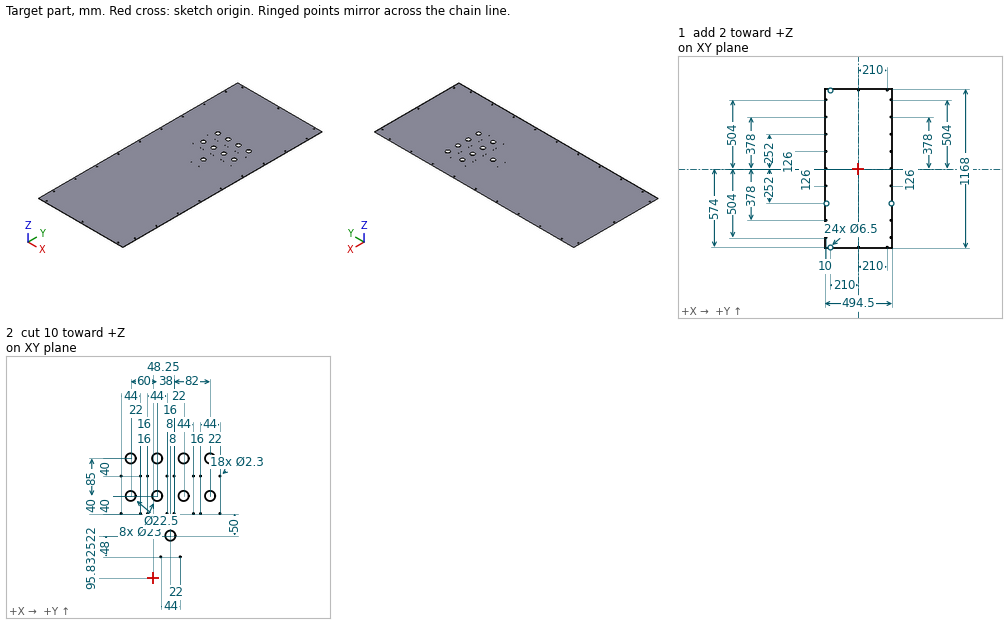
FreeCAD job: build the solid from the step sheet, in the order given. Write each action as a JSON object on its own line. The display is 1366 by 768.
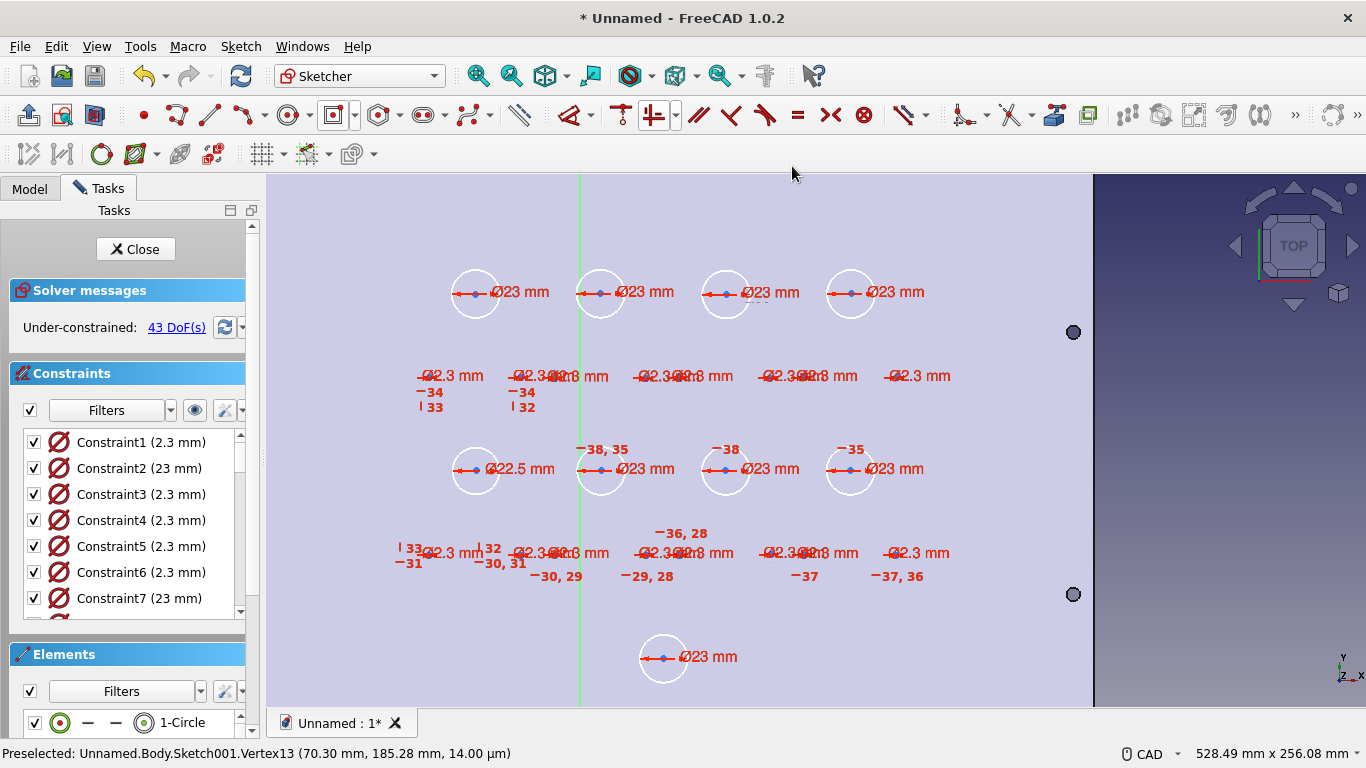
{"action": "left_click", "coordinate": [805, 555]}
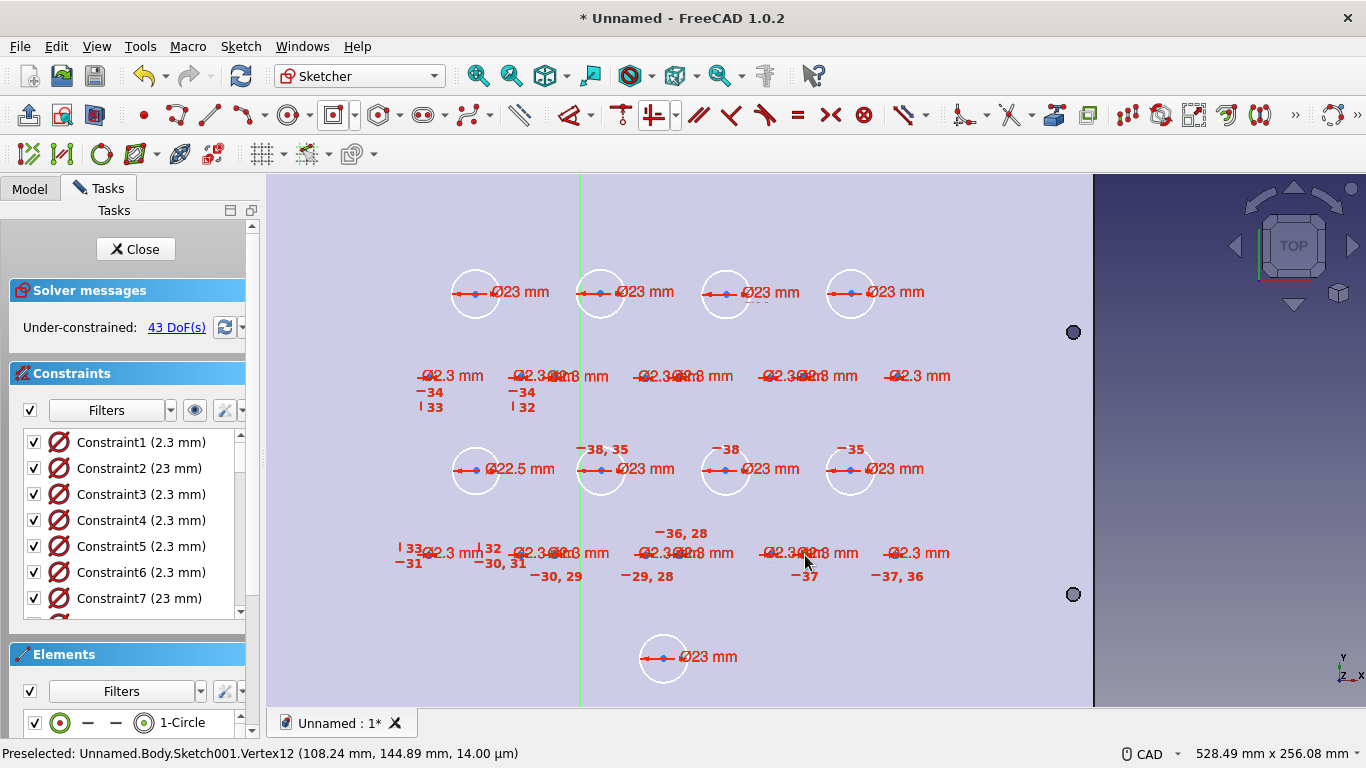
{"action": "left_click", "coordinate": [771, 555]}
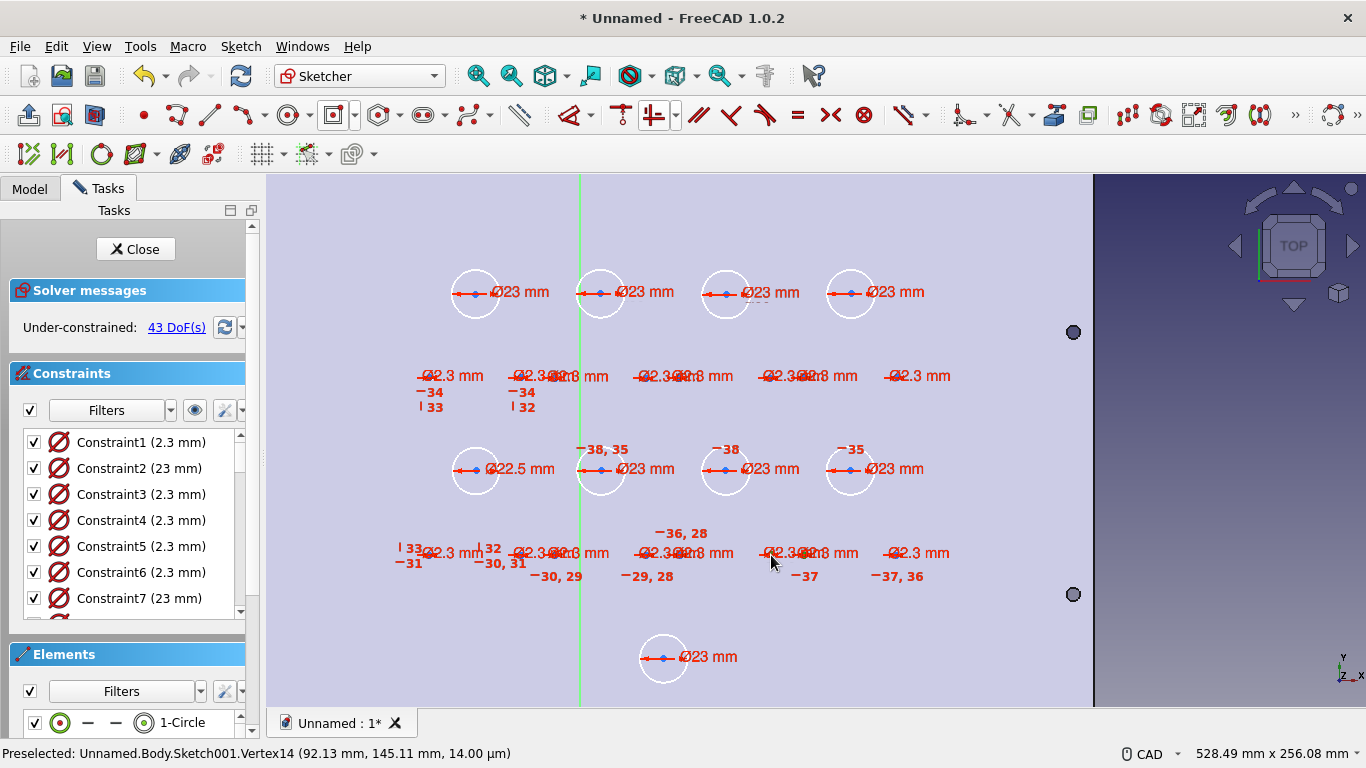
{"action": "left_click", "coordinate": [676, 116]}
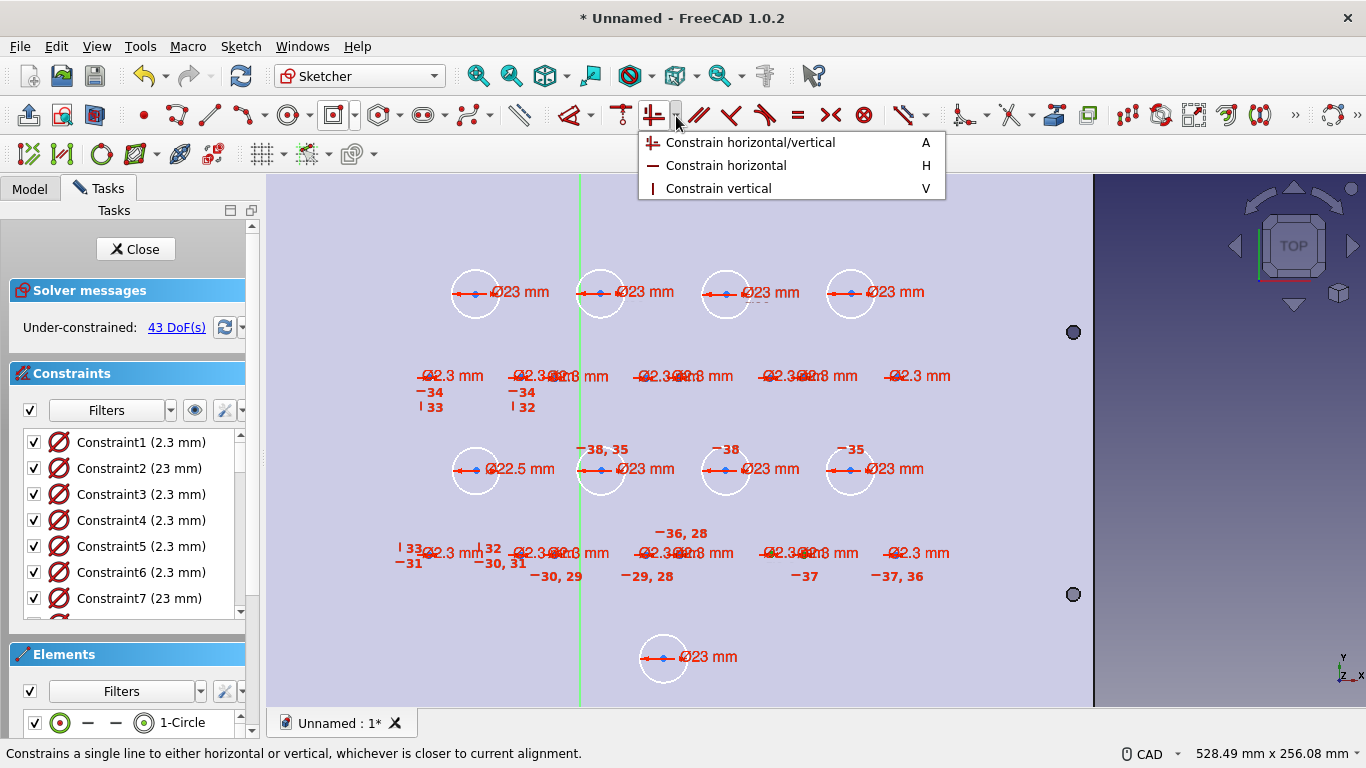
{"action": "left_click", "coordinate": [792, 166]}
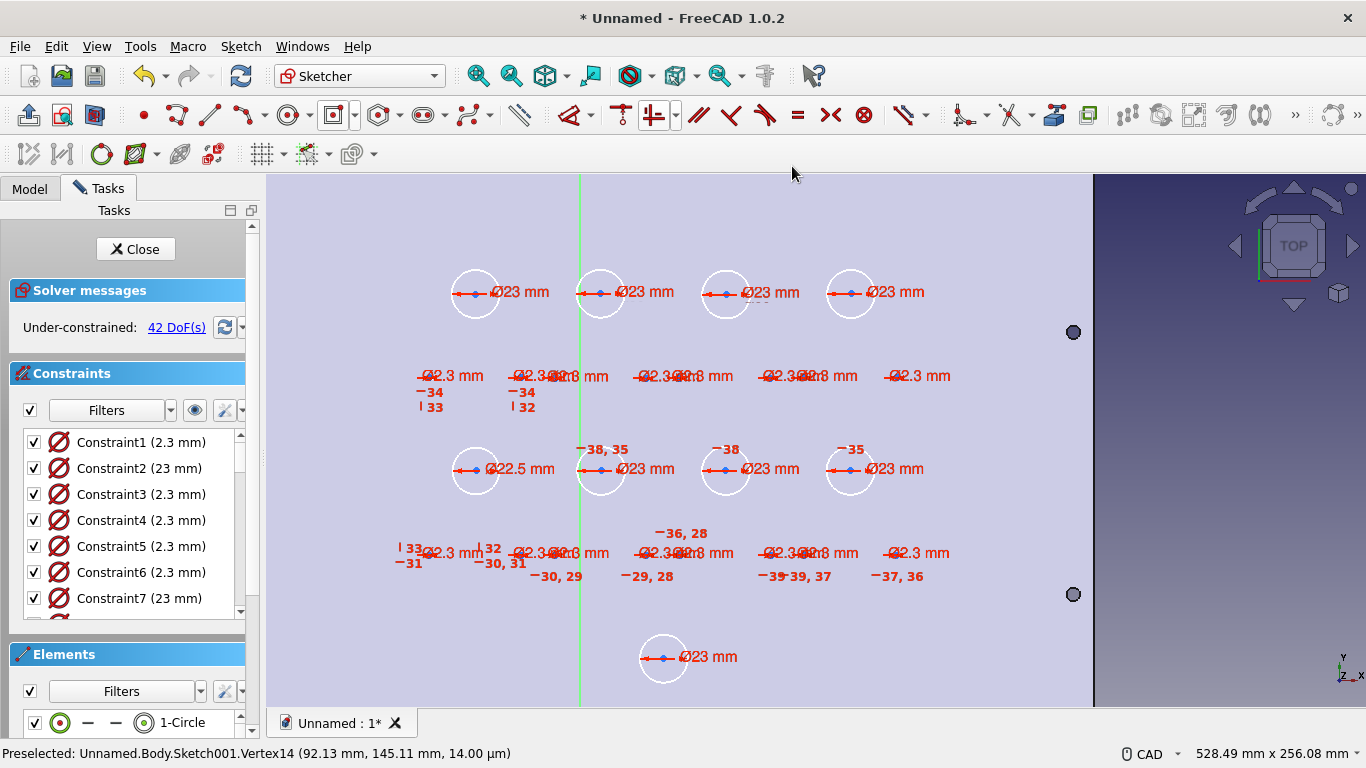
{"action": "left_click", "coordinate": [896, 555]}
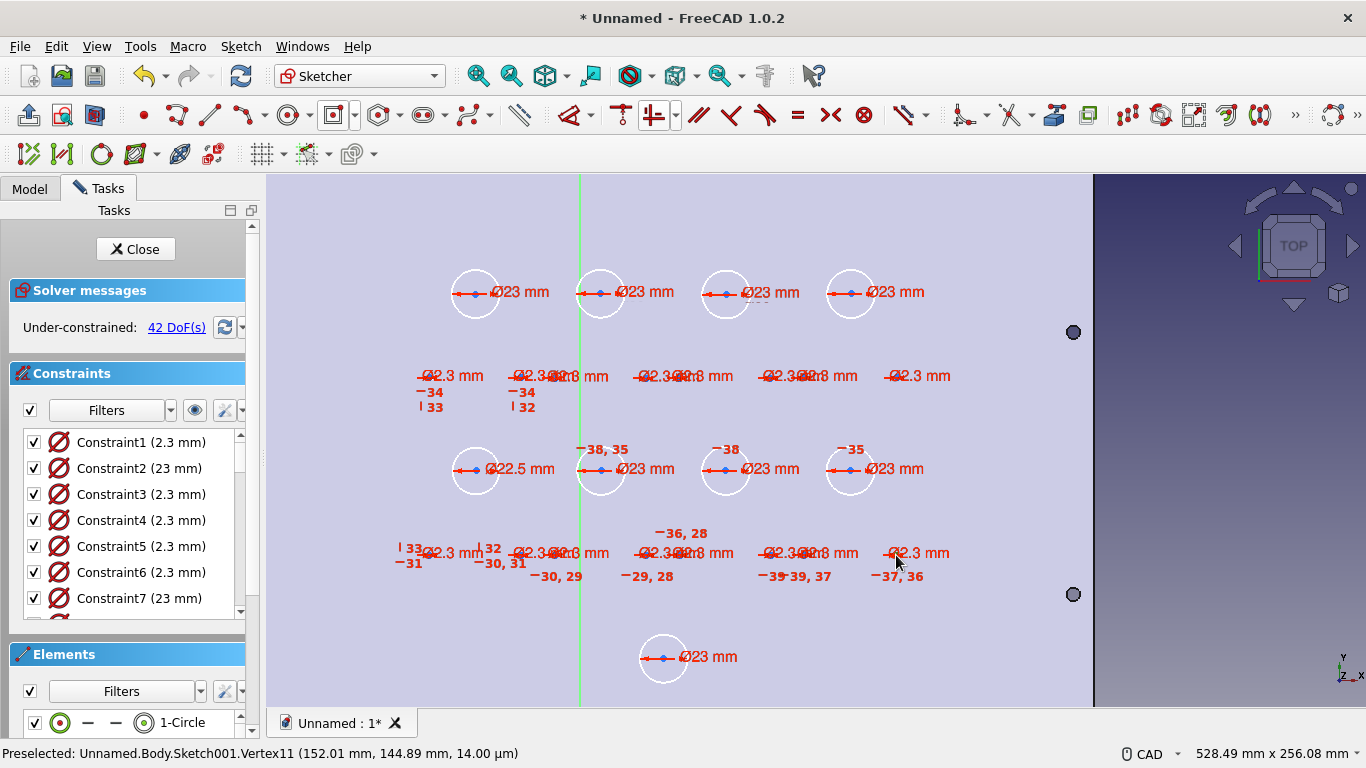
{"action": "left_click", "coordinate": [897, 378]}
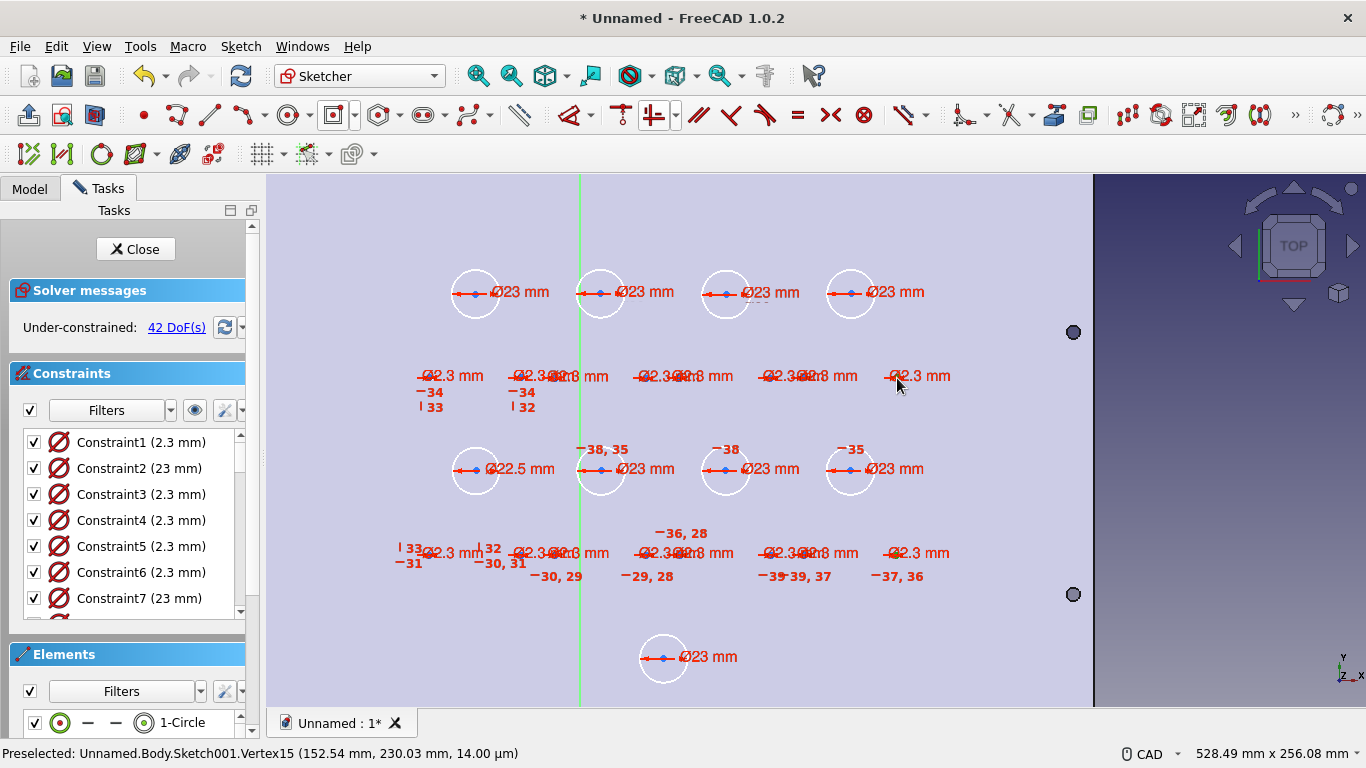
{"action": "left_click", "coordinate": [676, 116]}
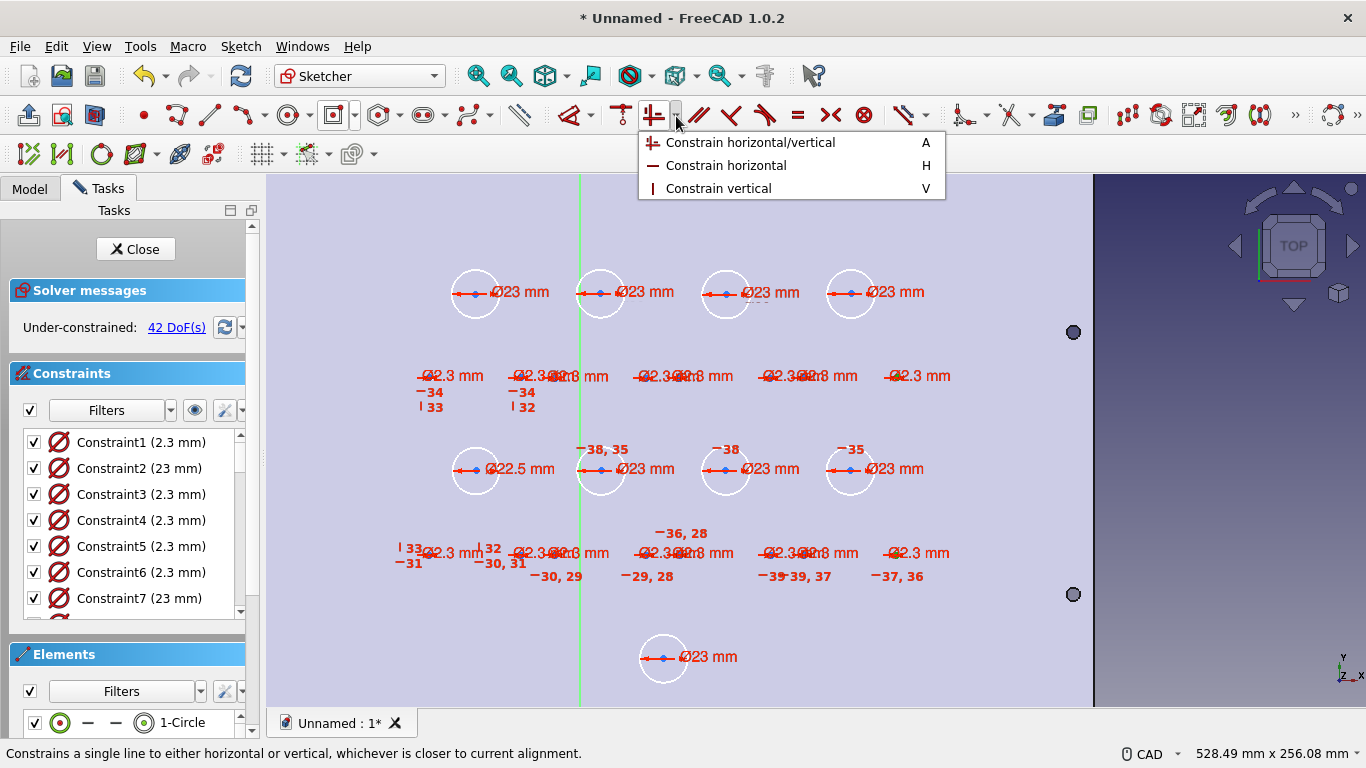
{"action": "left_click", "coordinate": [792, 188]}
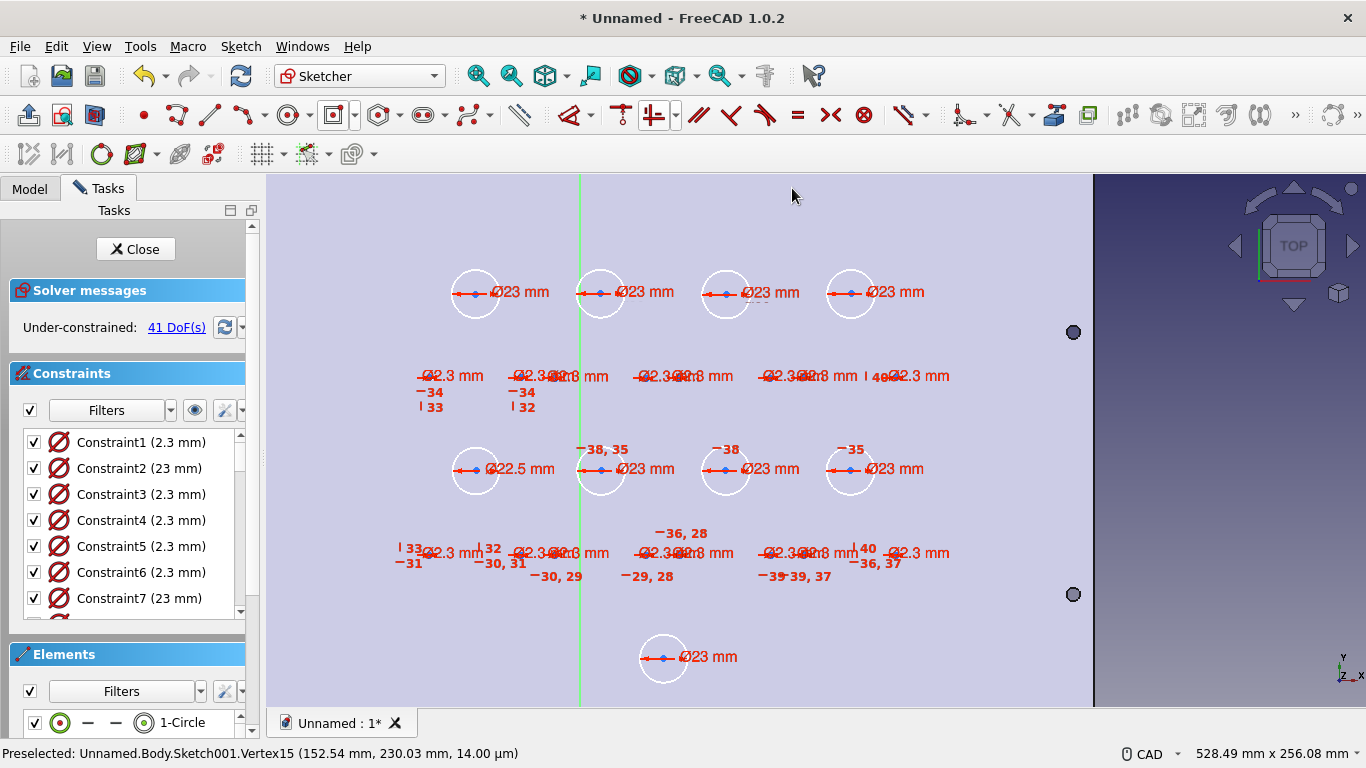
{"action": "left_click", "coordinate": [805, 555]}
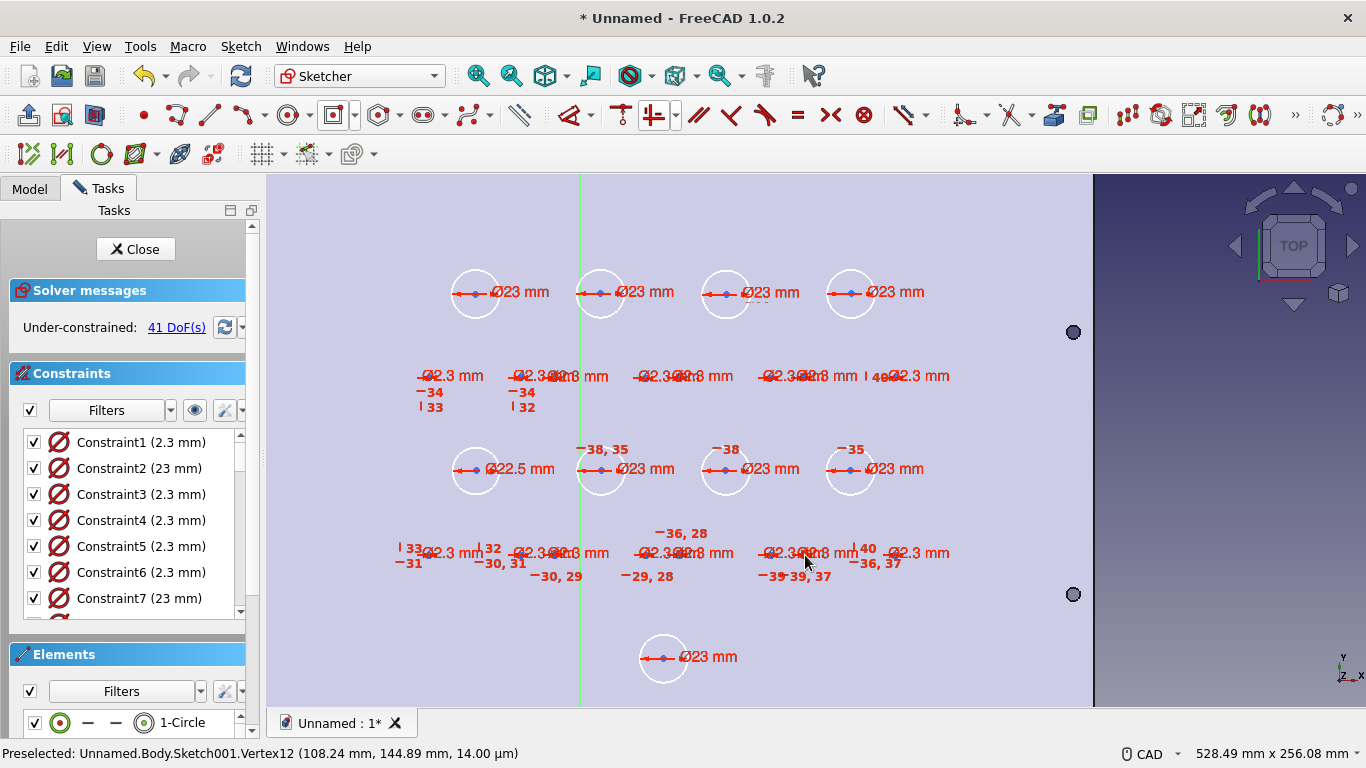
{"action": "left_click", "coordinate": [804, 378]}